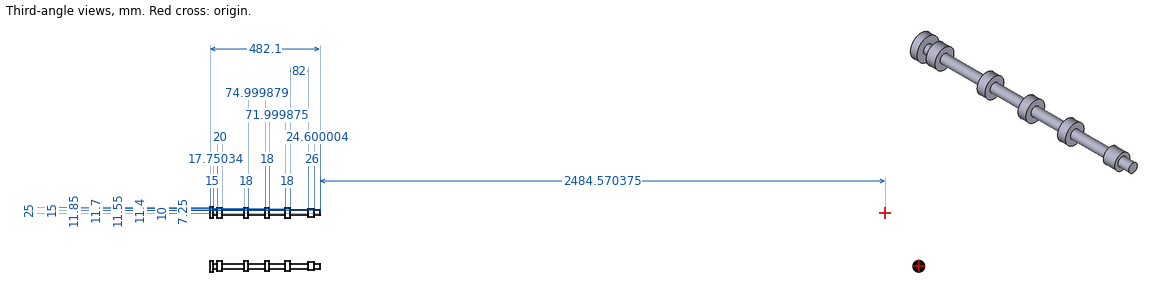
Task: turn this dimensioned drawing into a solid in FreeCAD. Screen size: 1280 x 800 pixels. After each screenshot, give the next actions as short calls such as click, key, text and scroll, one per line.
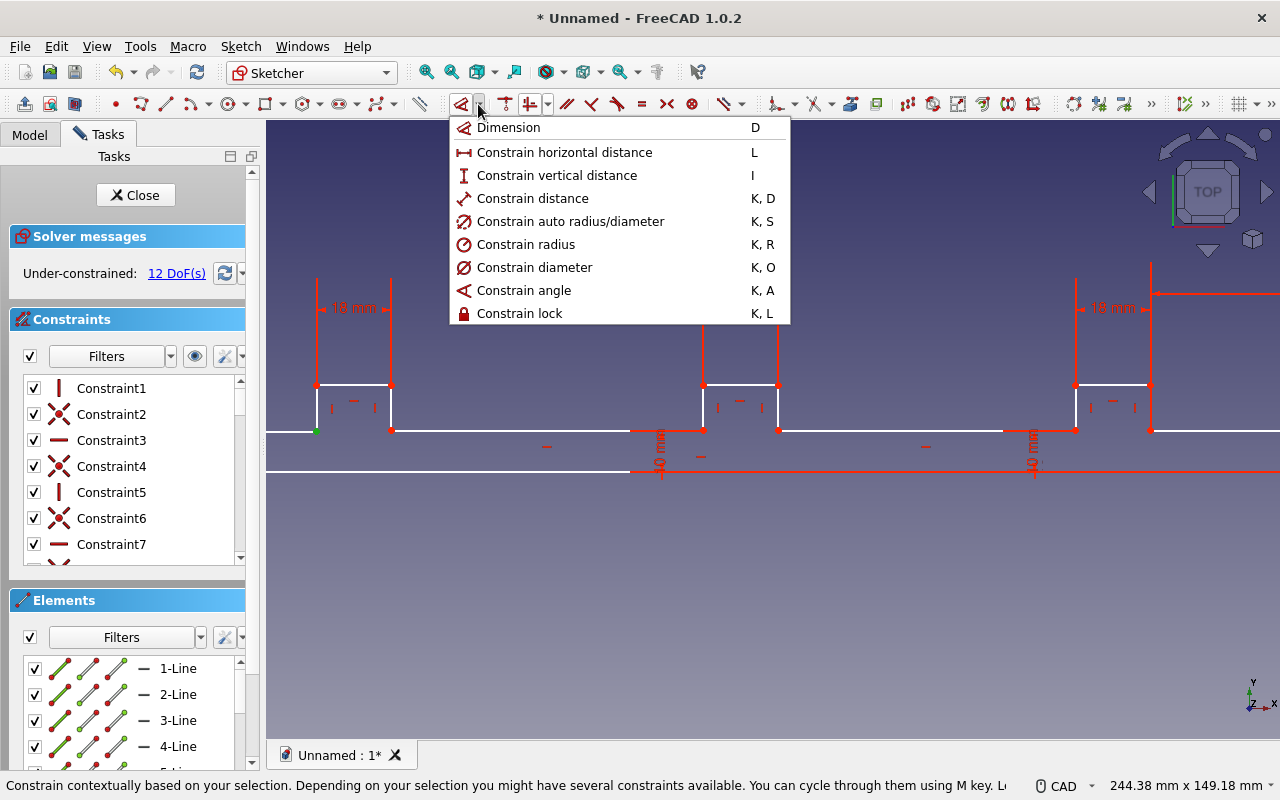
click(620, 176)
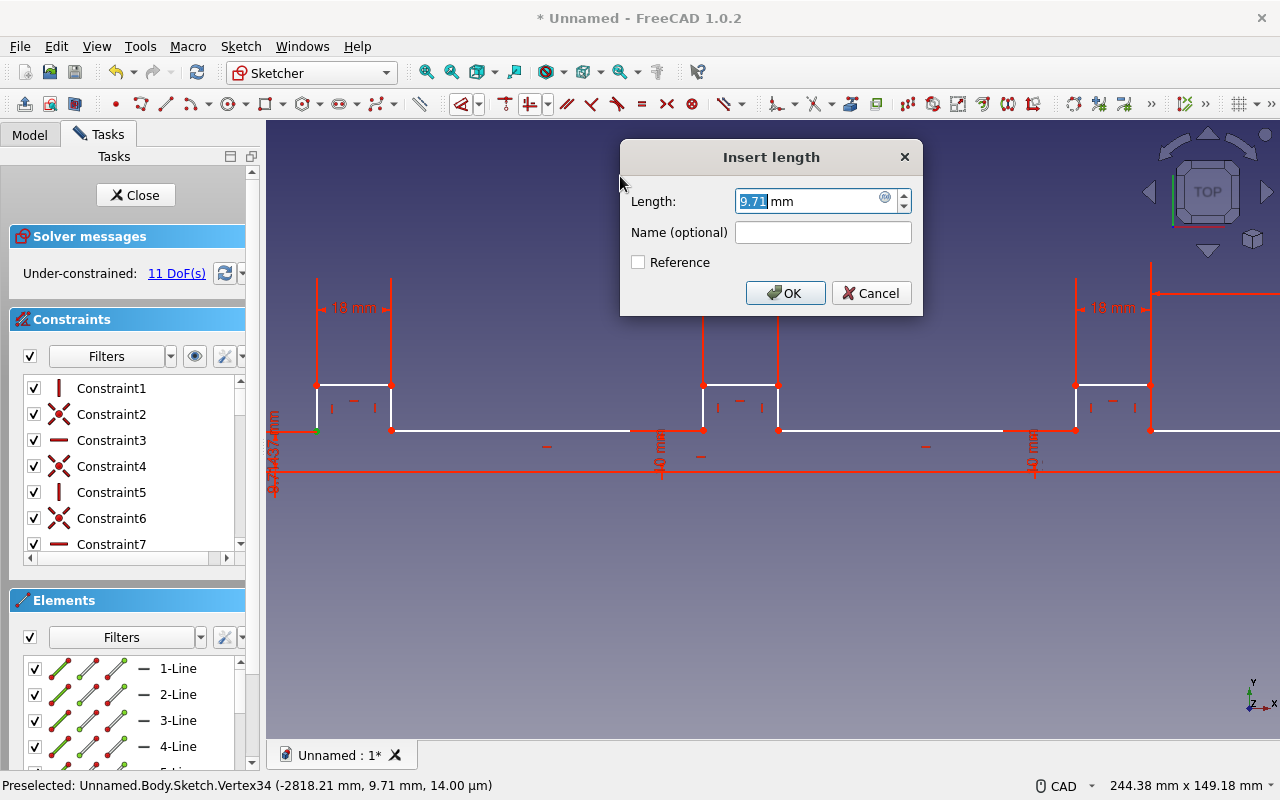
text(10)
key(Return)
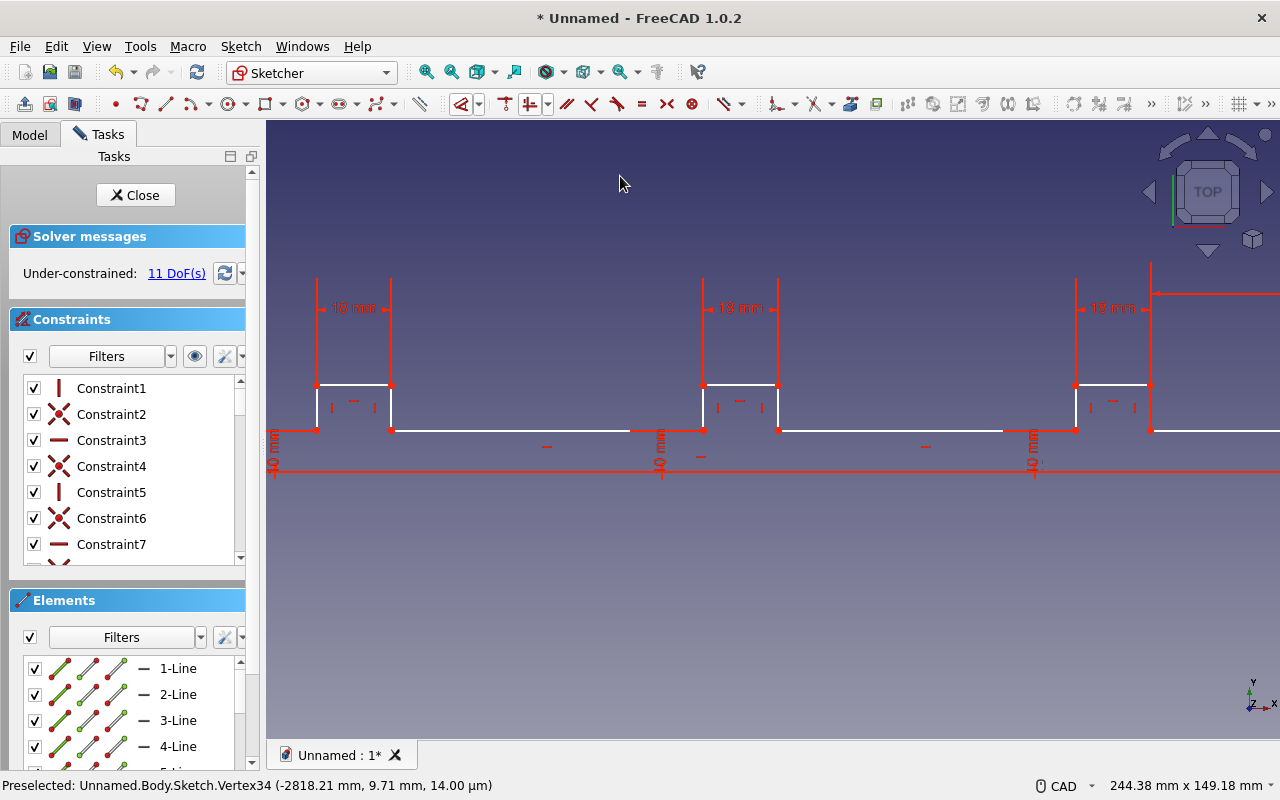
scroll(706, 433, down, 6)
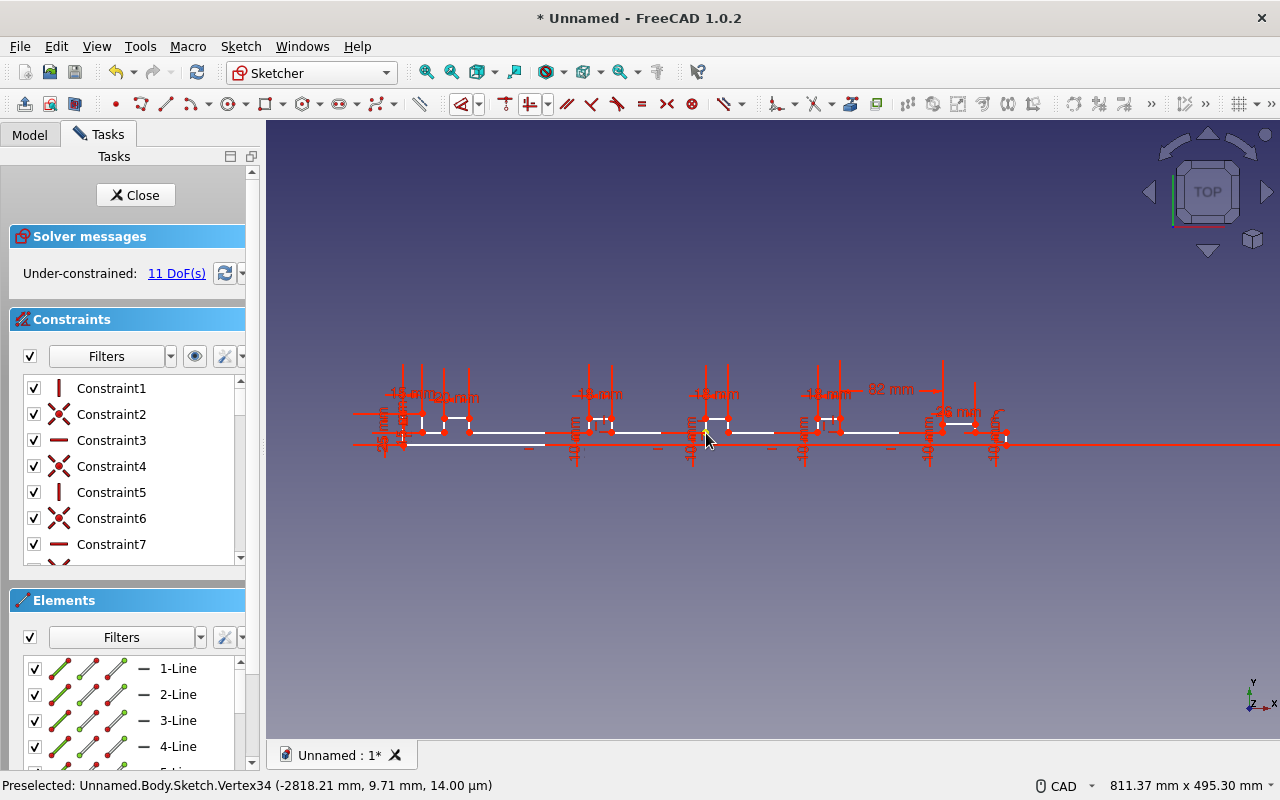
scroll(975, 429, up, 8)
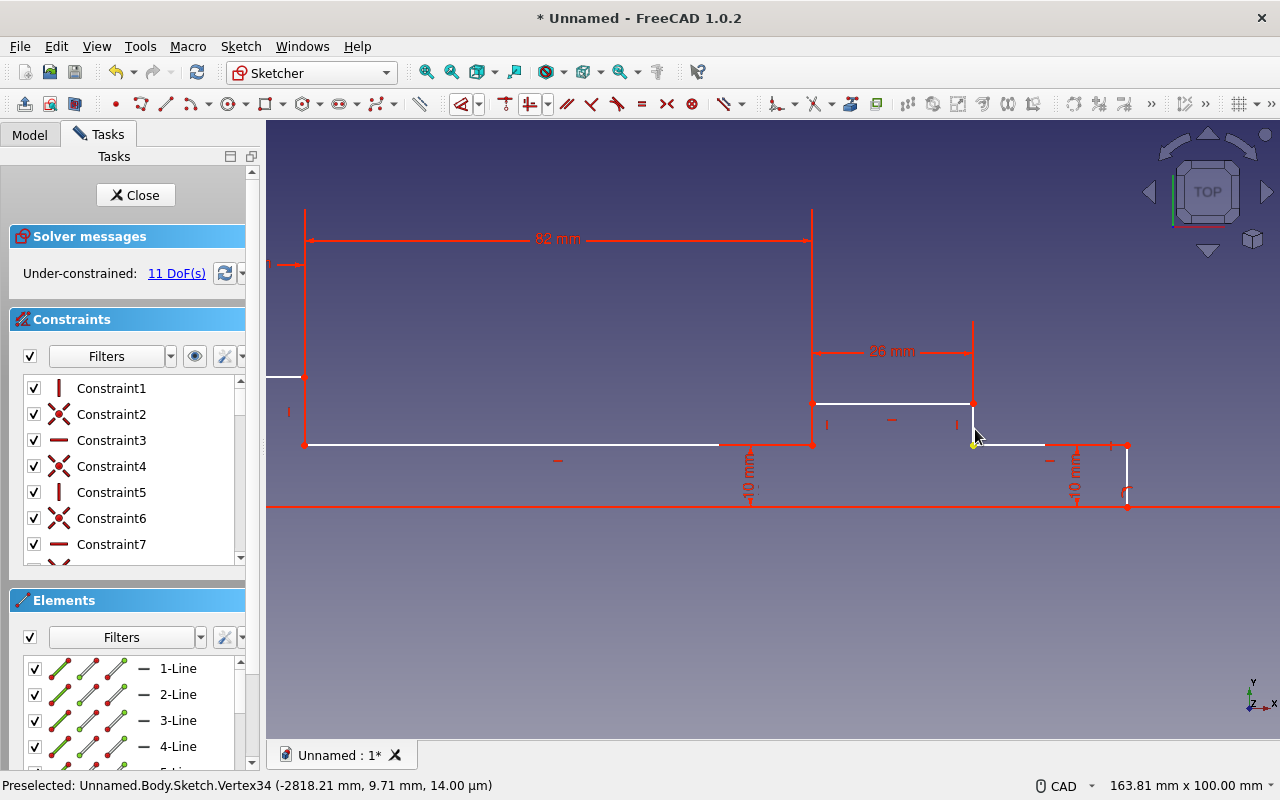
click(973, 429)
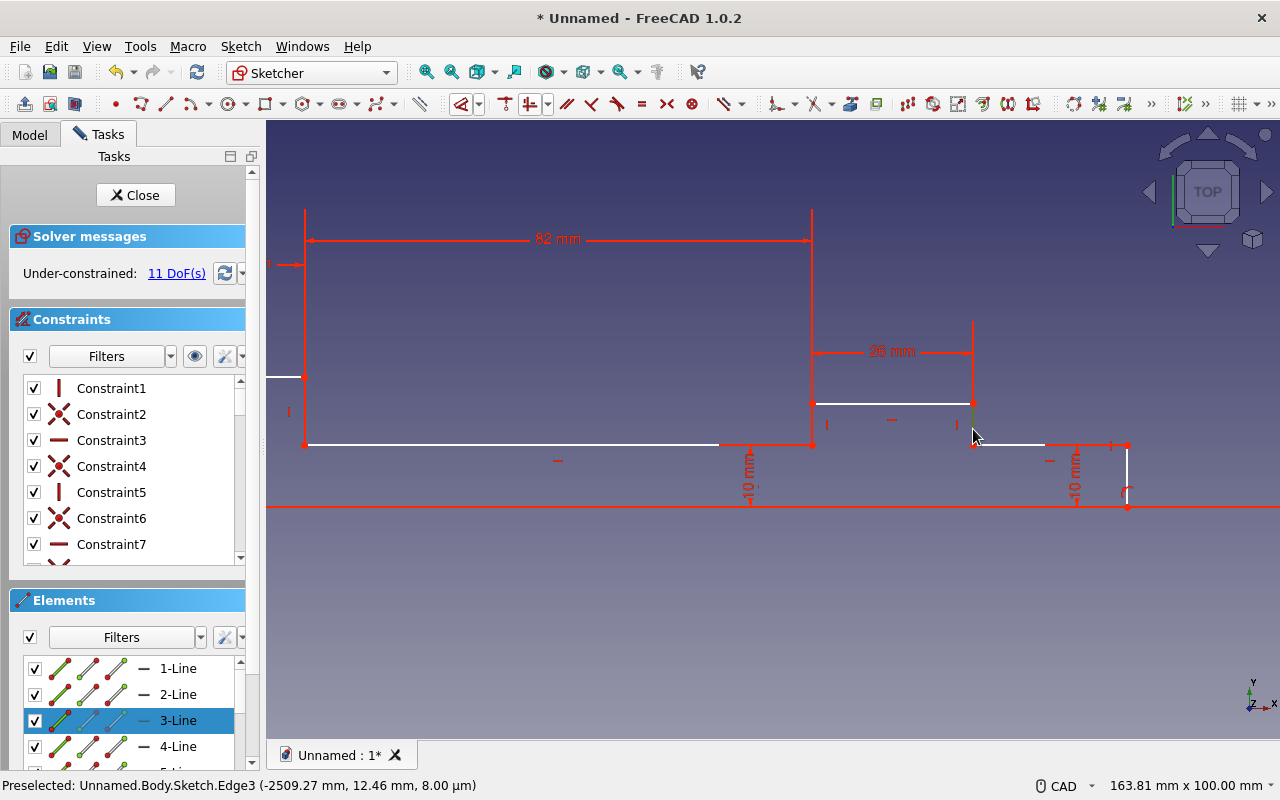
key(i)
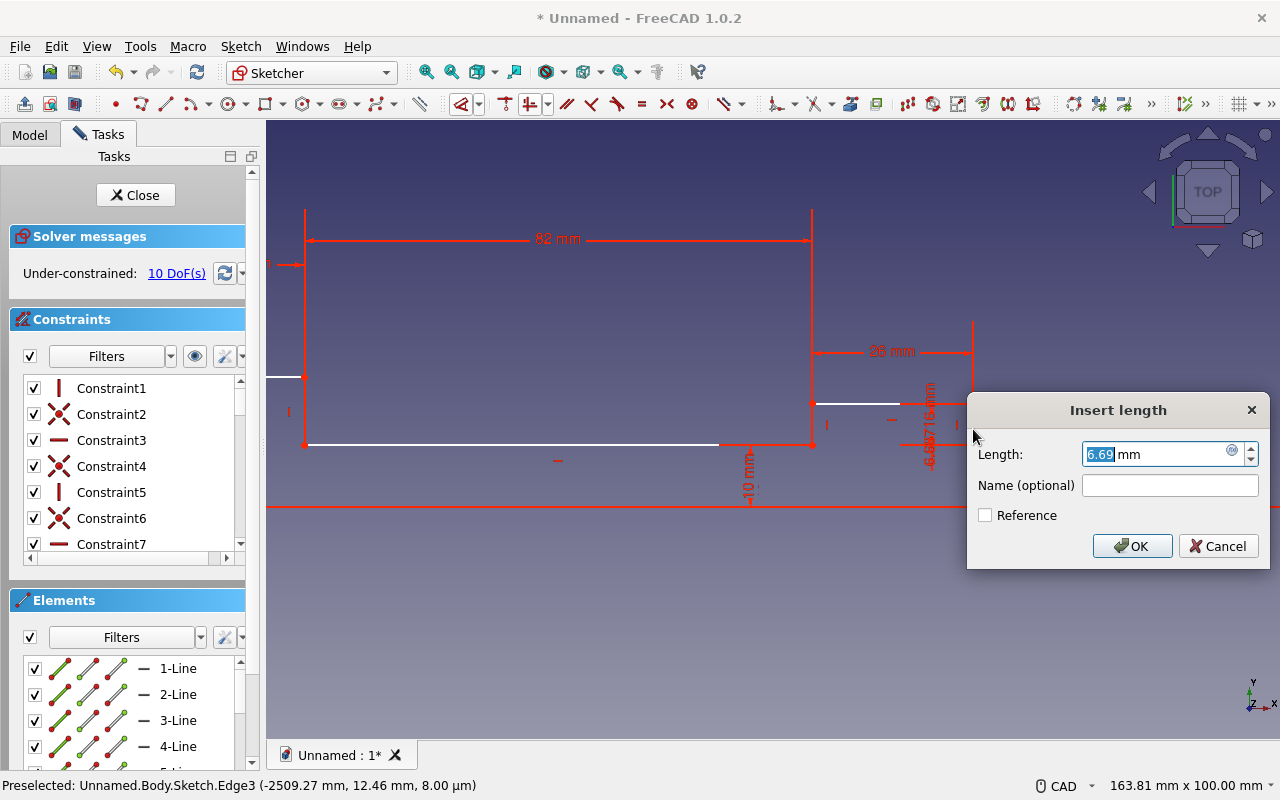
text(7.25)
key(Return)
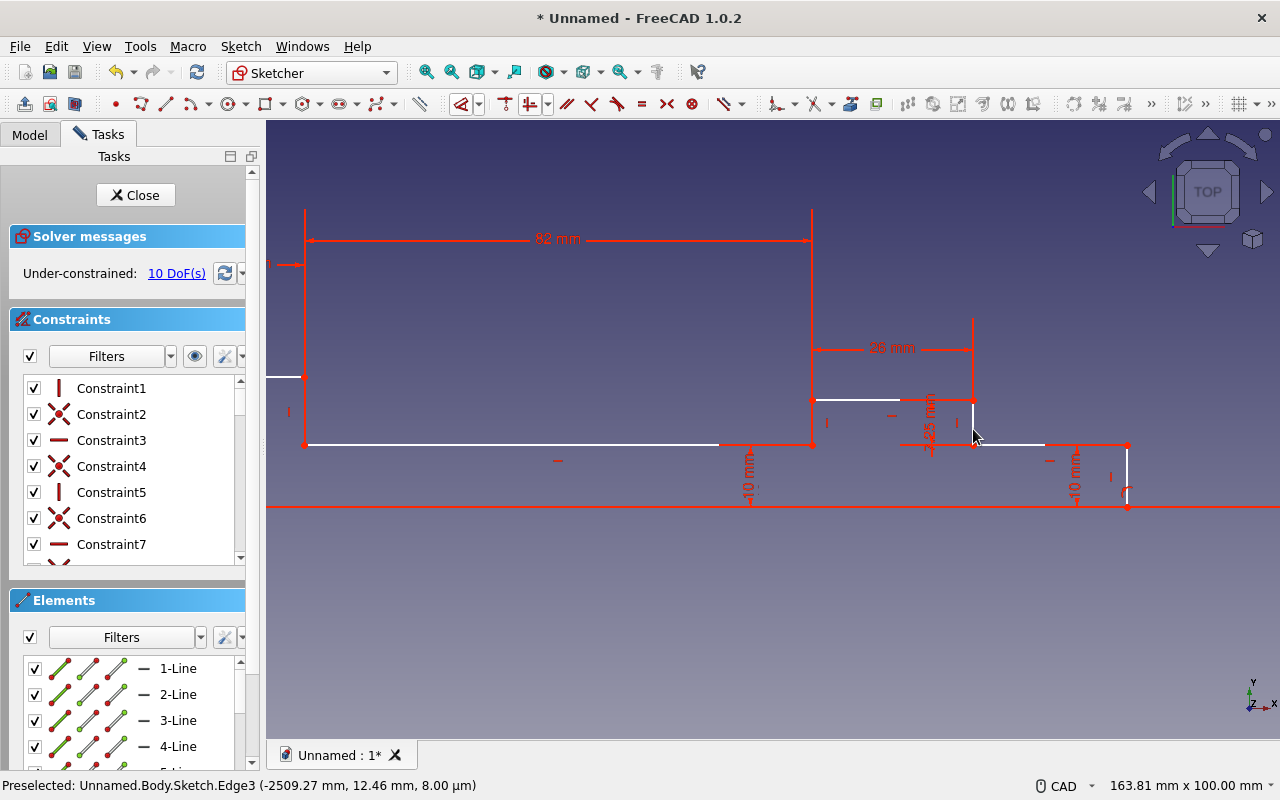
click(305, 425)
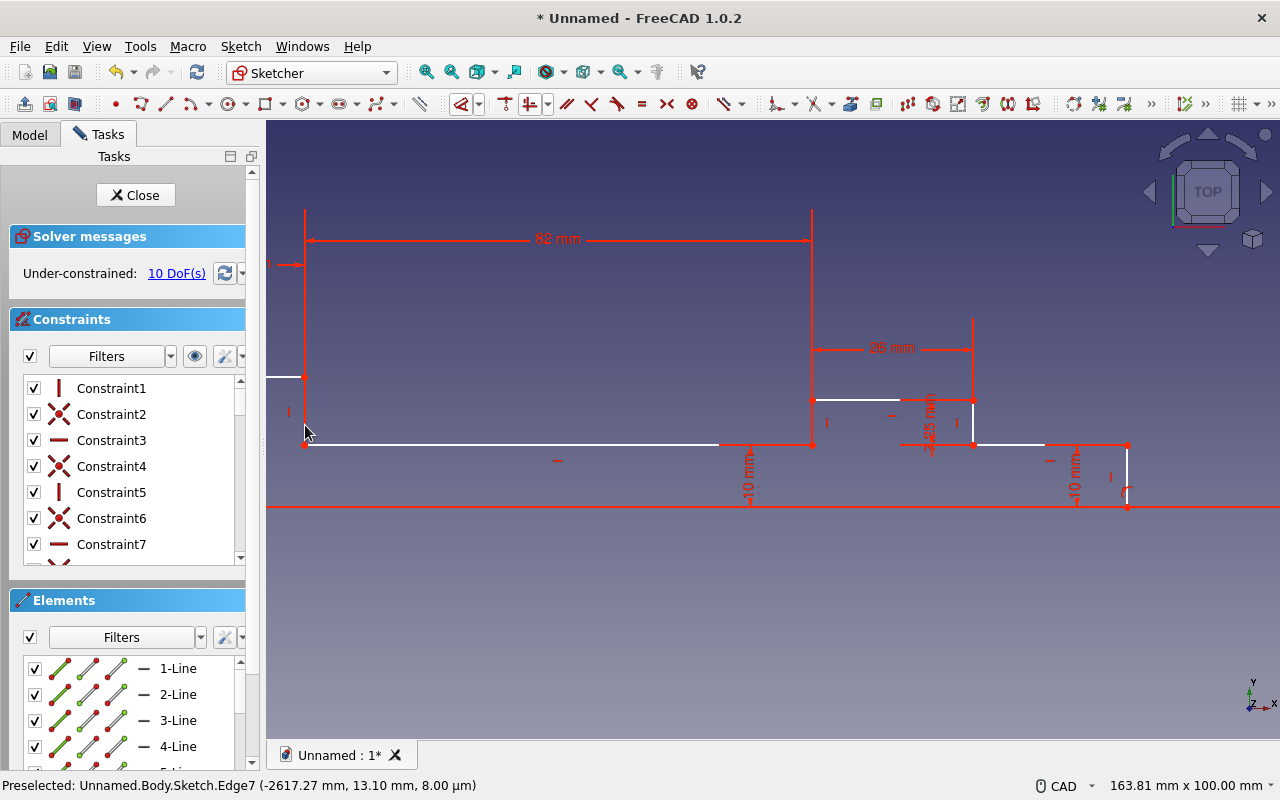
key(i)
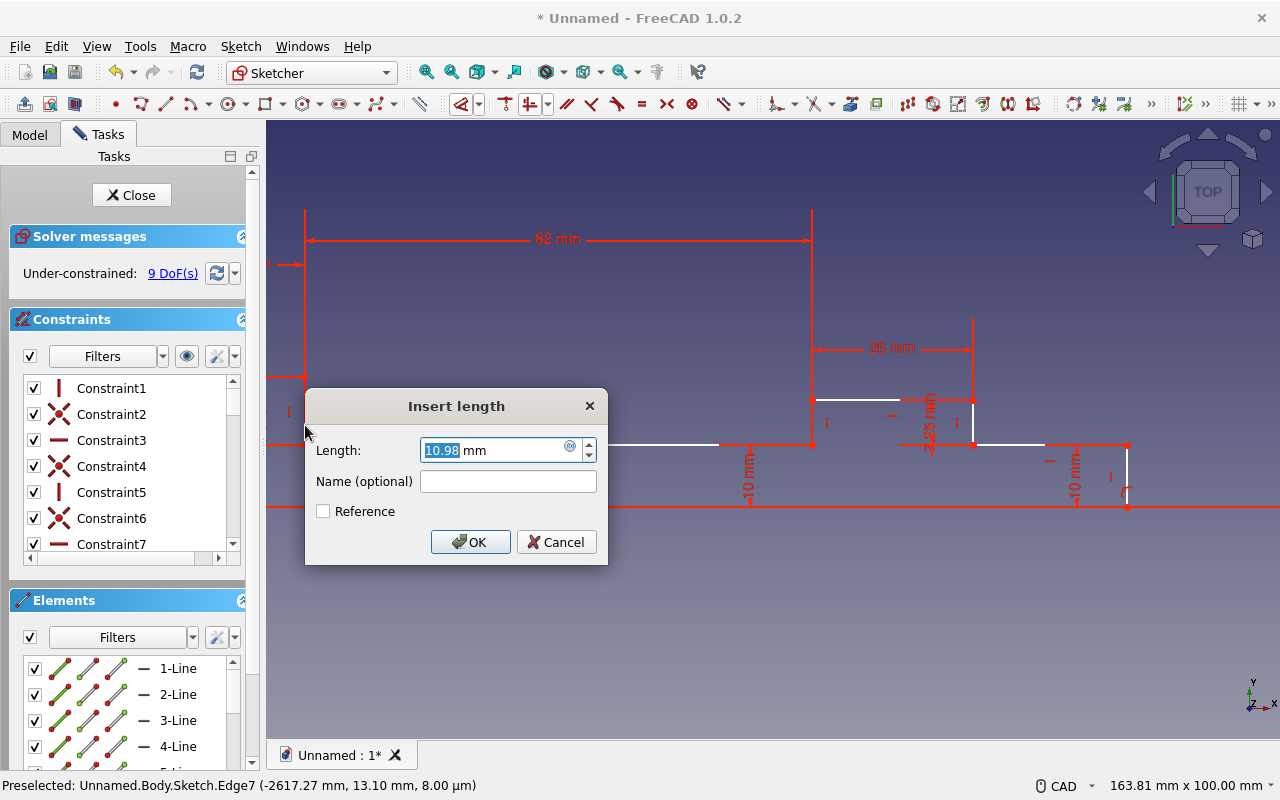
text(11.4)
key(Return)